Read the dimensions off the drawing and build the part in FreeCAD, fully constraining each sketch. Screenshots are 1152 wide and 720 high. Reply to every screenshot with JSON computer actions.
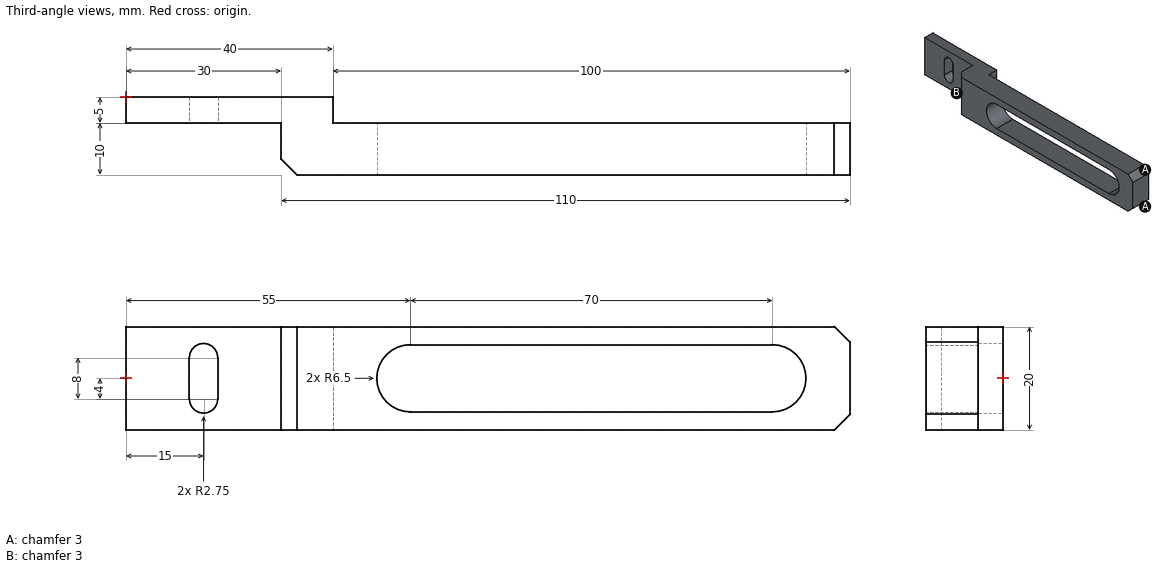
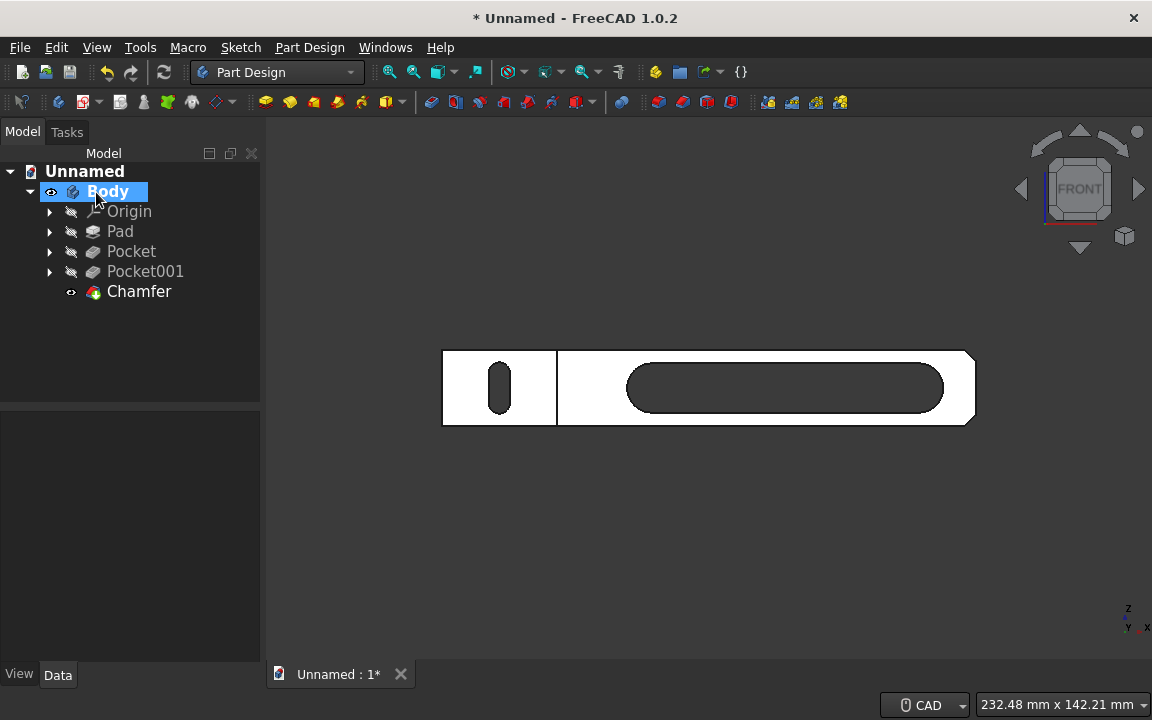
{"action": "left_click", "coordinate": [557, 387]}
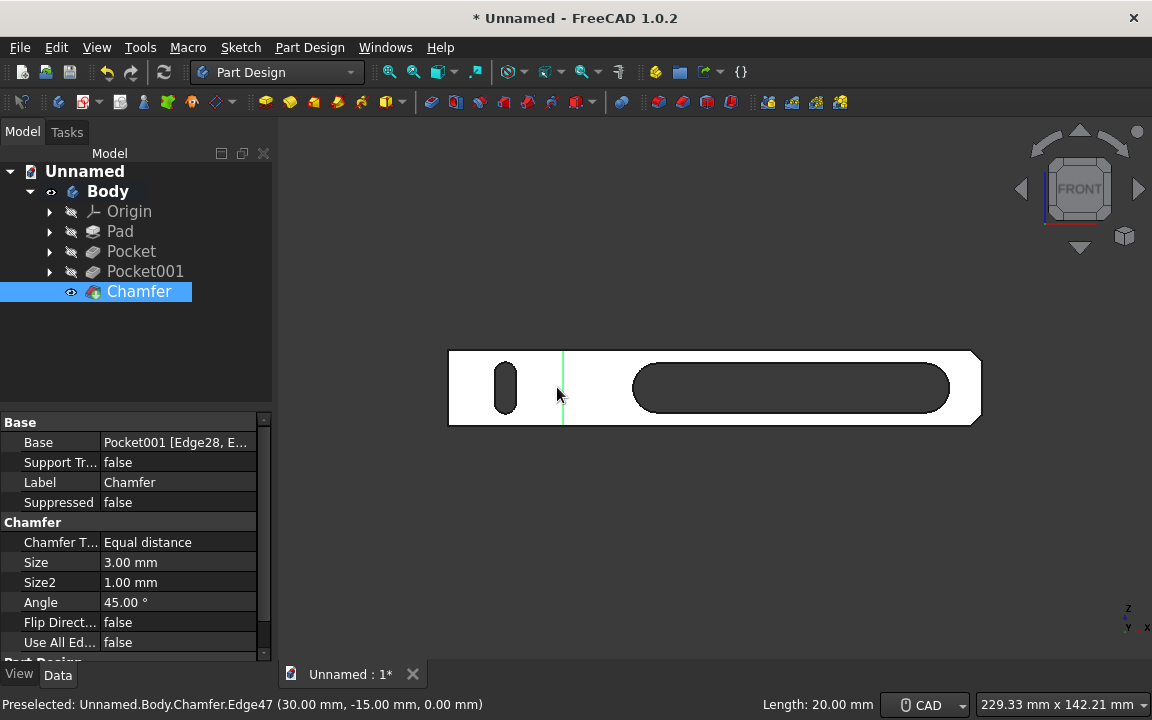
{"action": "left_click", "coordinate": [684, 102]}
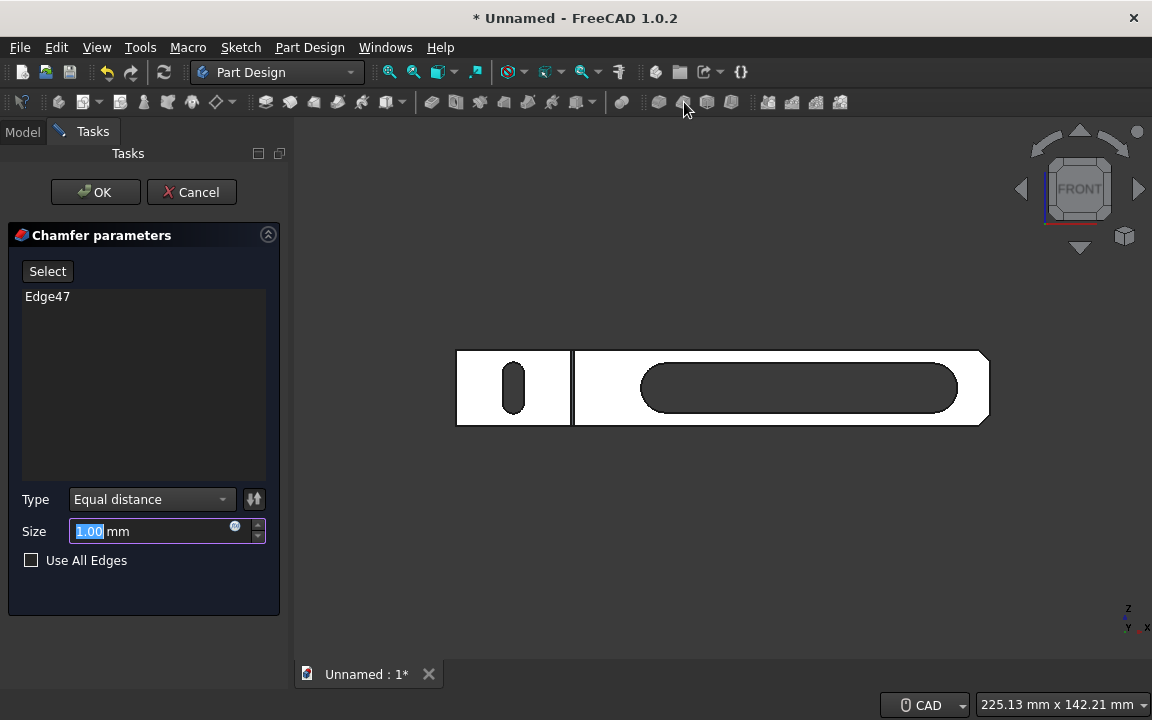
{"action": "type", "text": "3"}
{"action": "key", "text": "Tab"}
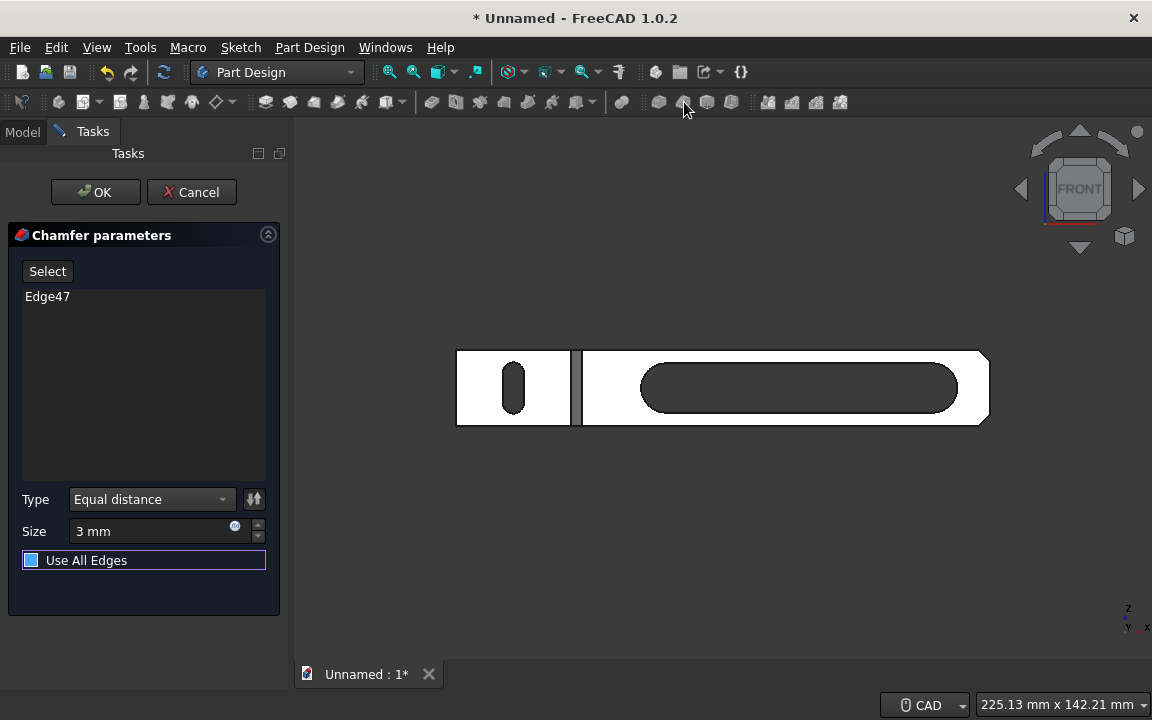
{"action": "left_click", "coordinate": [96, 192]}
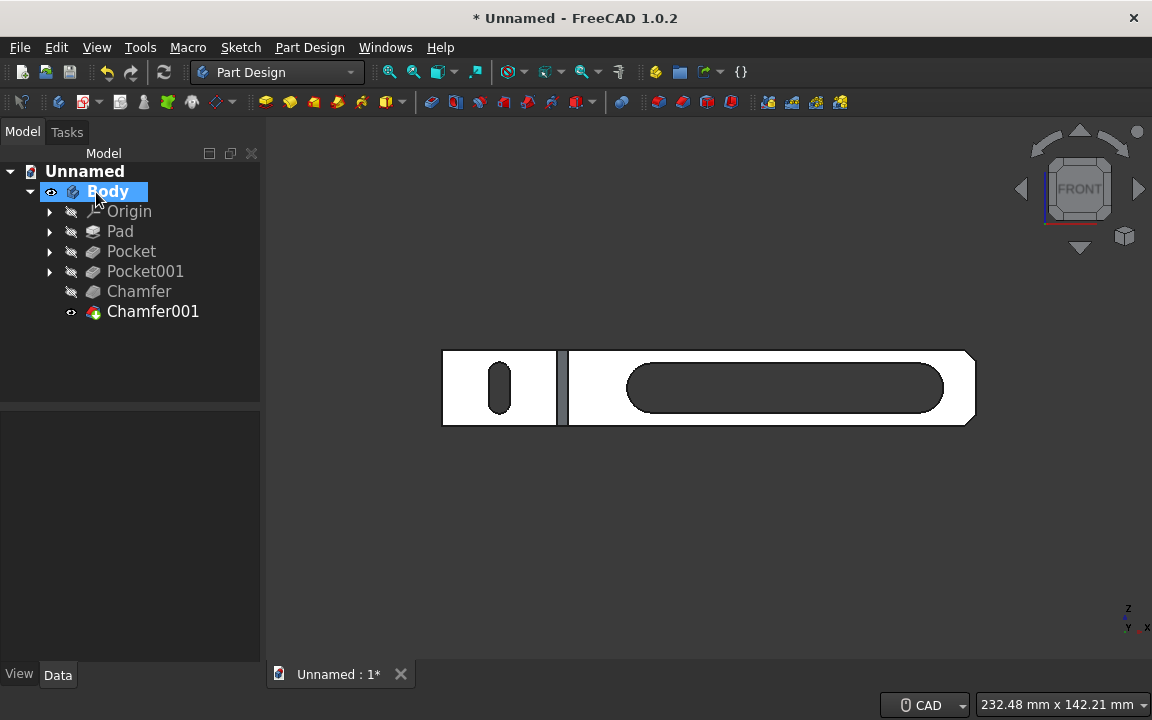
{"action": "key", "text": "0"}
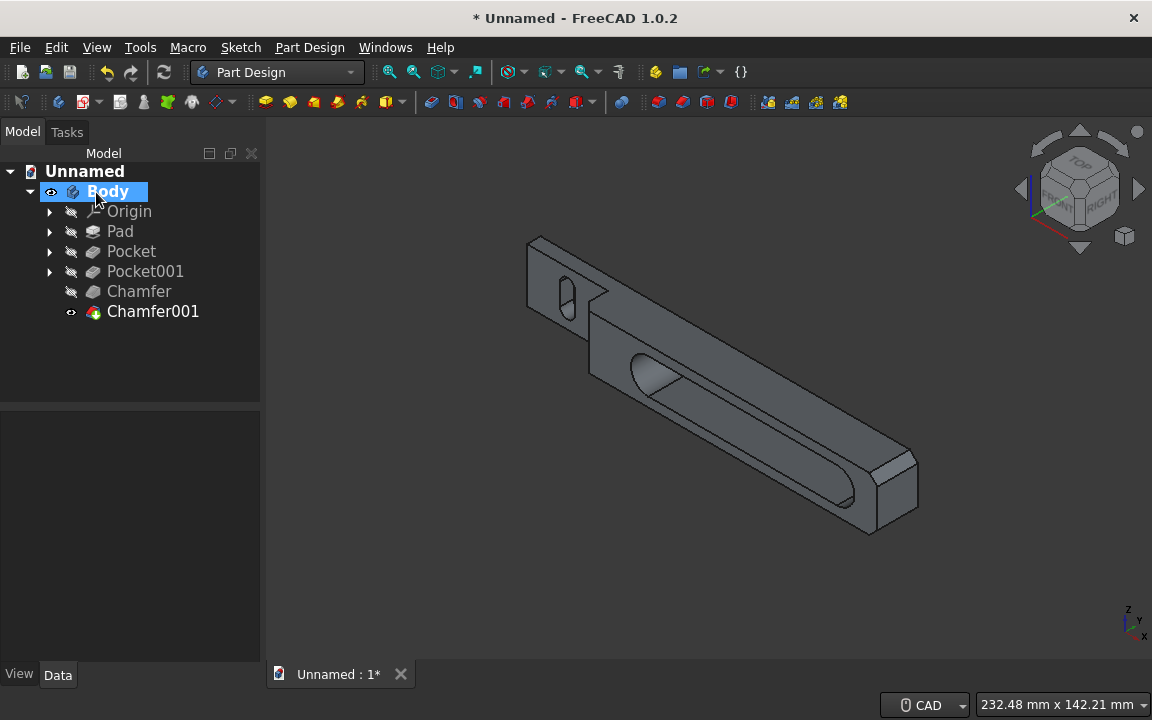
{"action": "left_click", "coordinate": [863, 445]}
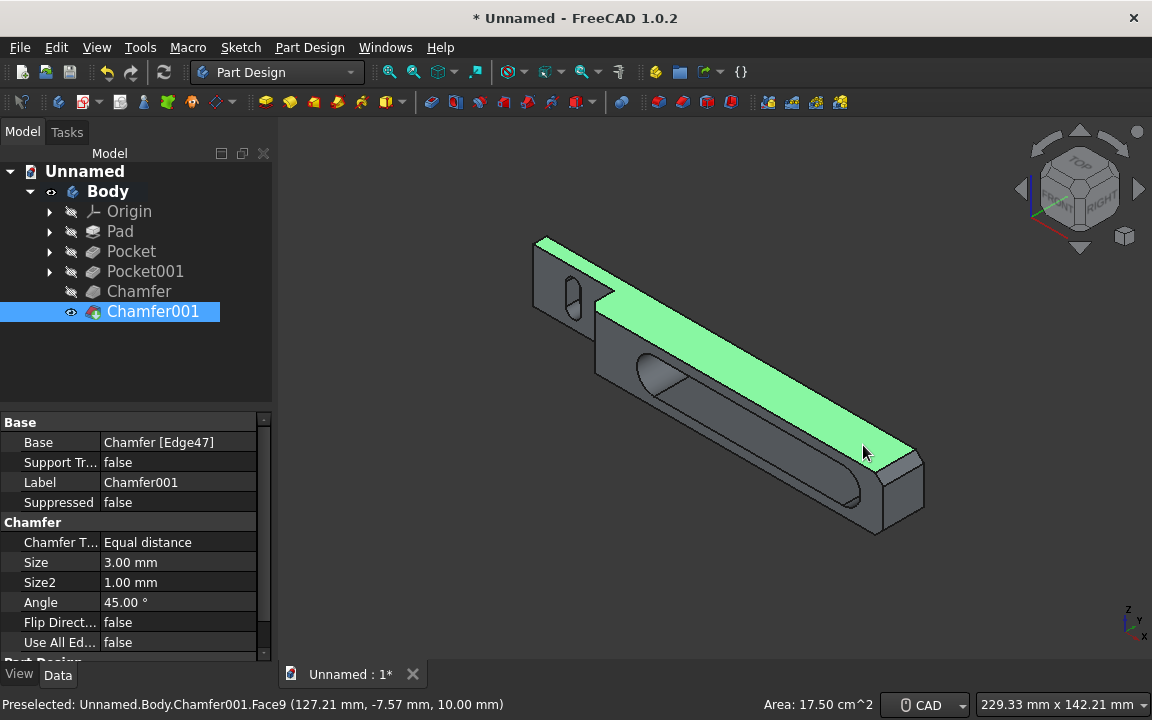
{"action": "left_click", "coordinate": [84, 102]}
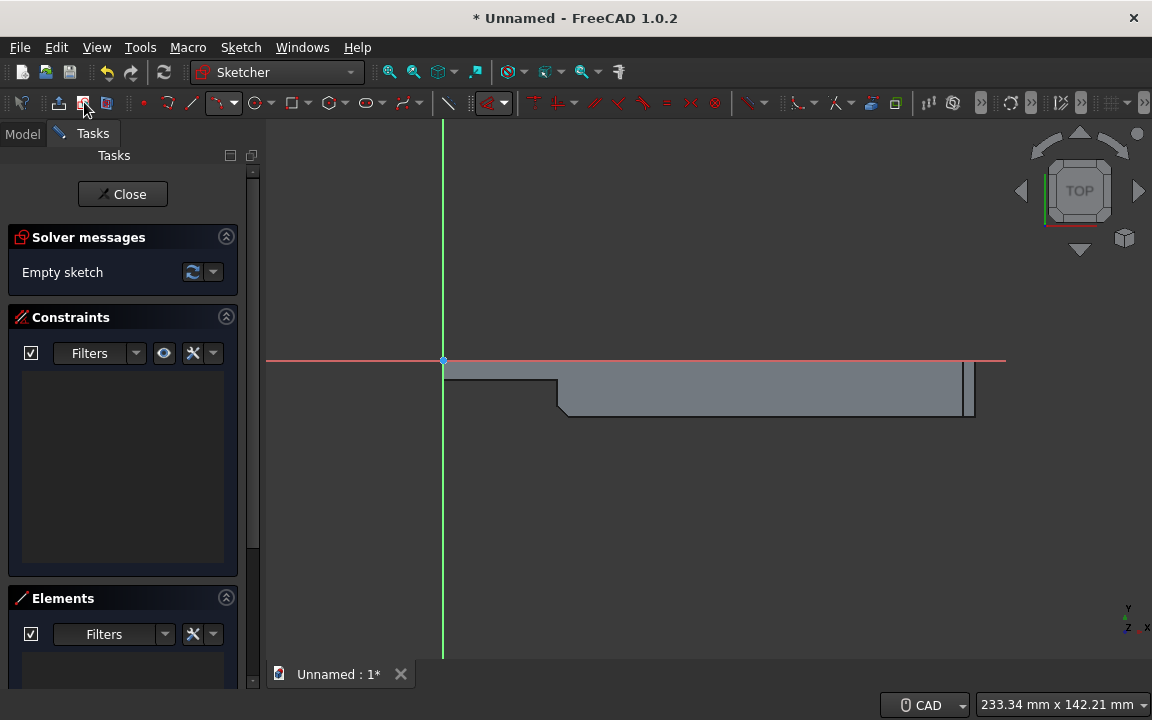
{"action": "scroll", "coordinate": [331, 475], "scroll_direction": "down", "scroll_amount": 1}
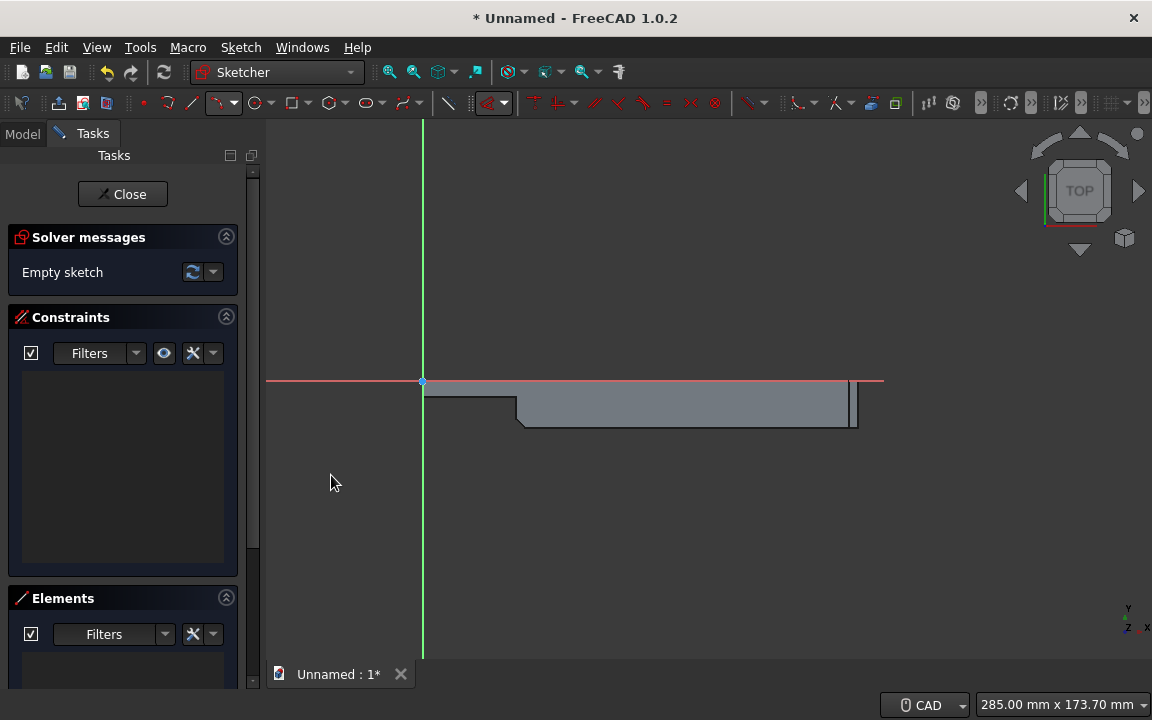
{"action": "left_click", "coordinate": [292, 104]}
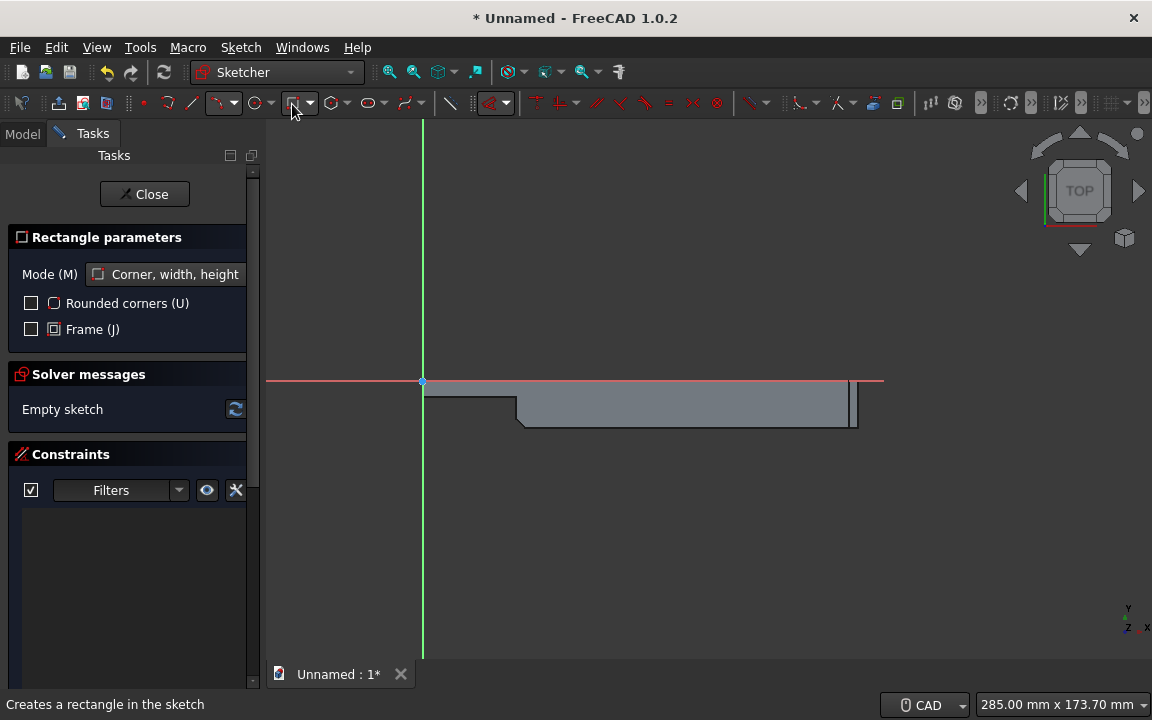
{"action": "left_click", "coordinate": [547, 381]}
{"action": "left_click", "coordinate": [858, 397]}
{"action": "key", "text": "Escape"}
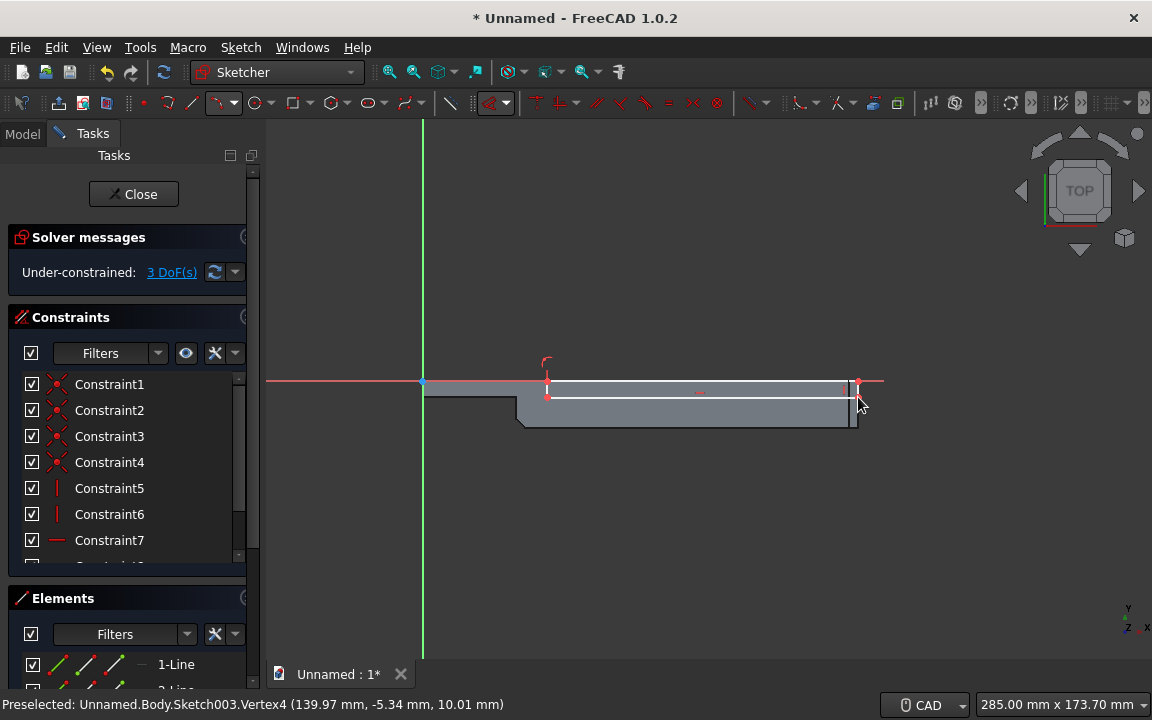
{"action": "scroll", "coordinate": [547, 390], "scroll_direction": "up", "scroll_amount": 5}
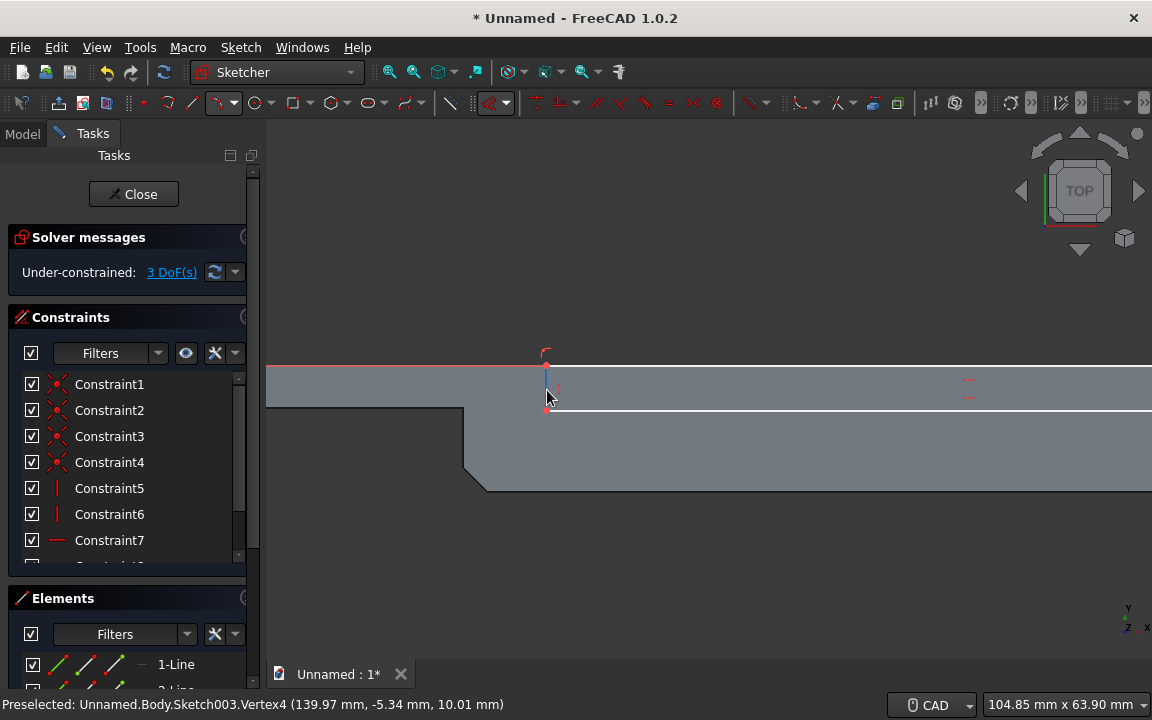
{"action": "left_click", "coordinate": [546, 388]}